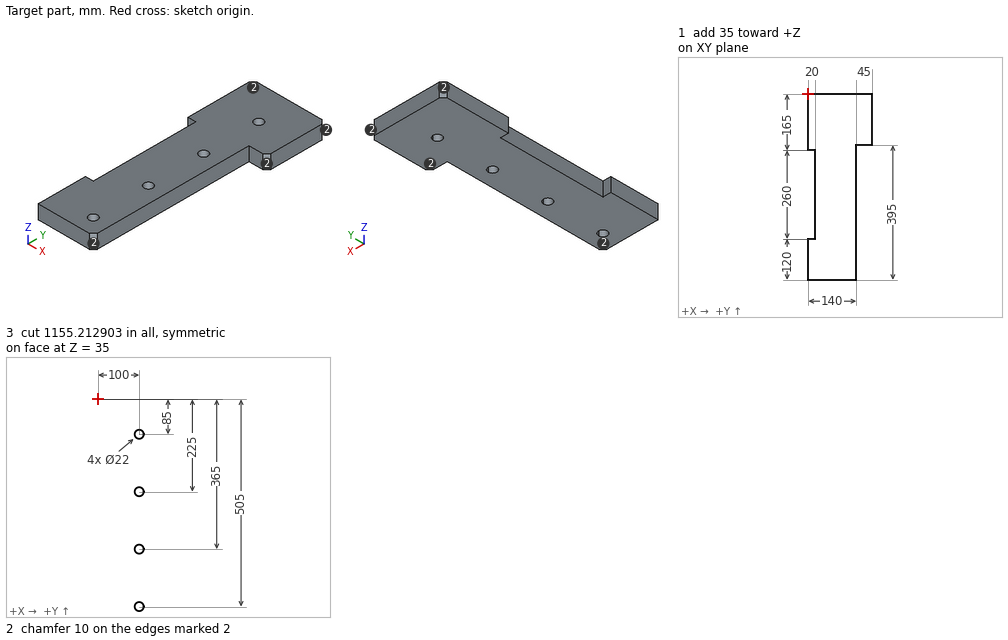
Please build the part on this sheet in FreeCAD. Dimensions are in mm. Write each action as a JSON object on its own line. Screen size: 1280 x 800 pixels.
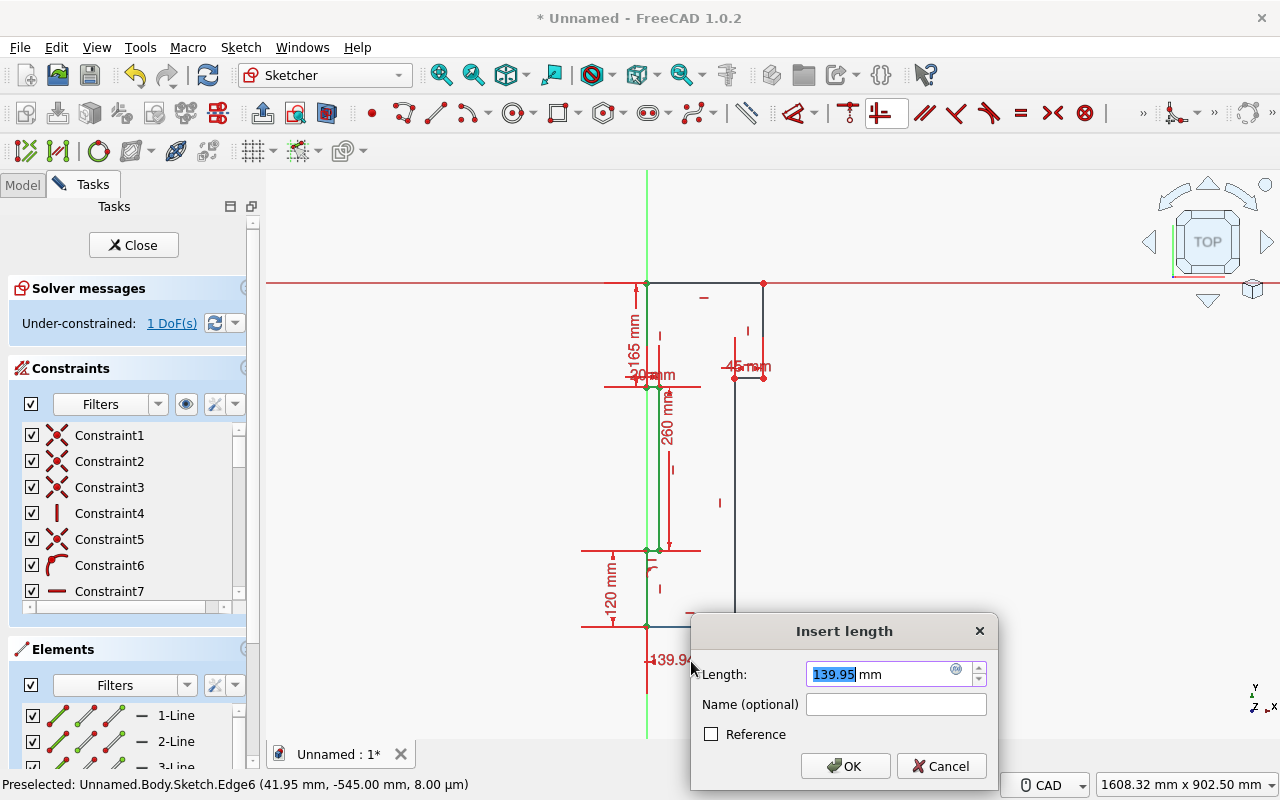
{"action": "type", "text": "140"}
{"action": "key", "text": "Return"}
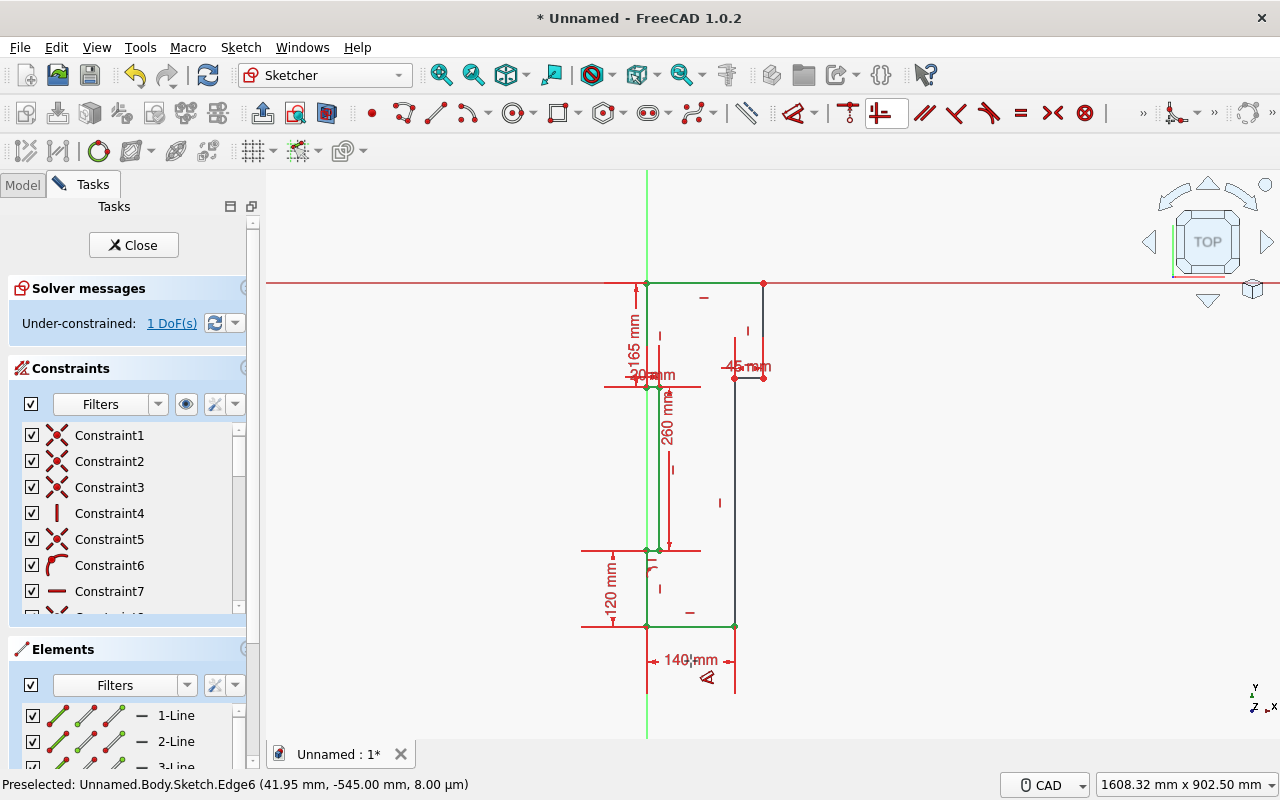
{"action": "left_click", "coordinate": [735, 552]}
{"action": "left_click", "coordinate": [769, 503]}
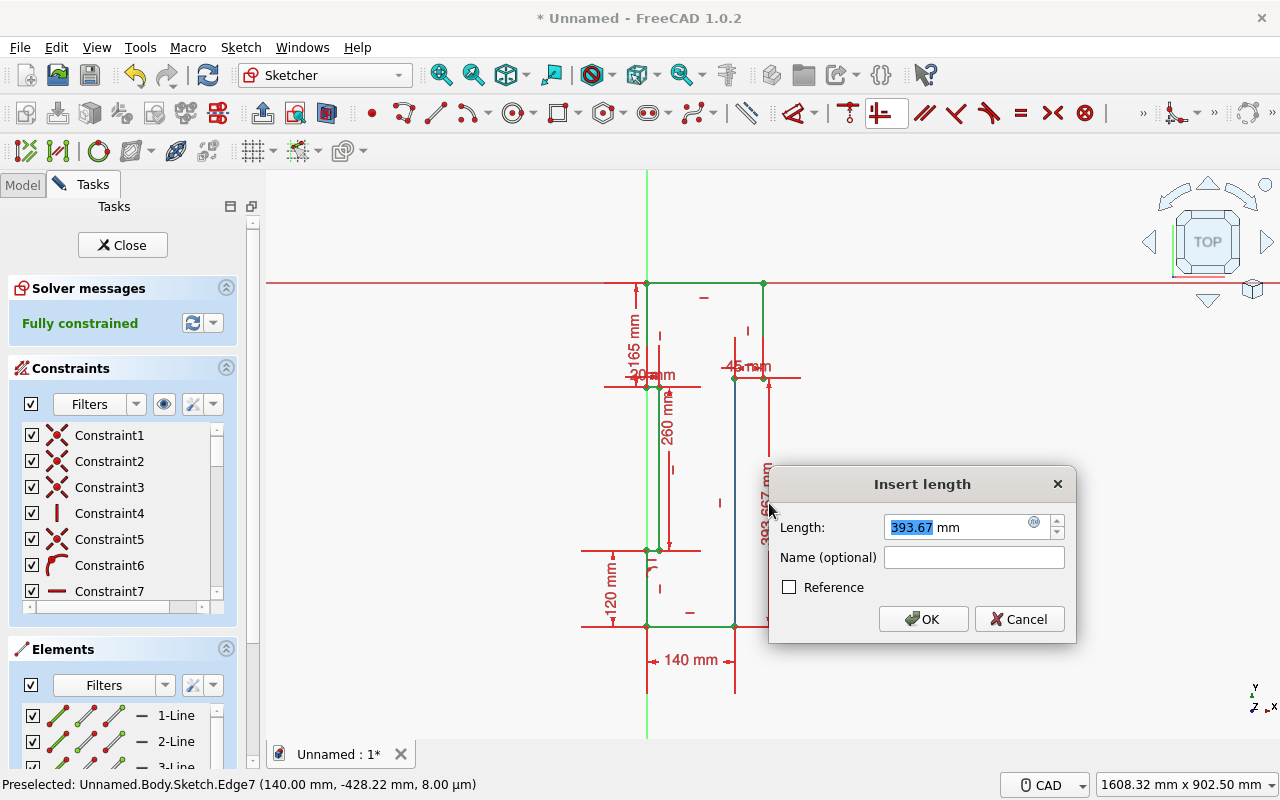
{"action": "type", "text": "395"}
{"action": "key", "text": "Return"}
{"action": "key", "text": "Escape"}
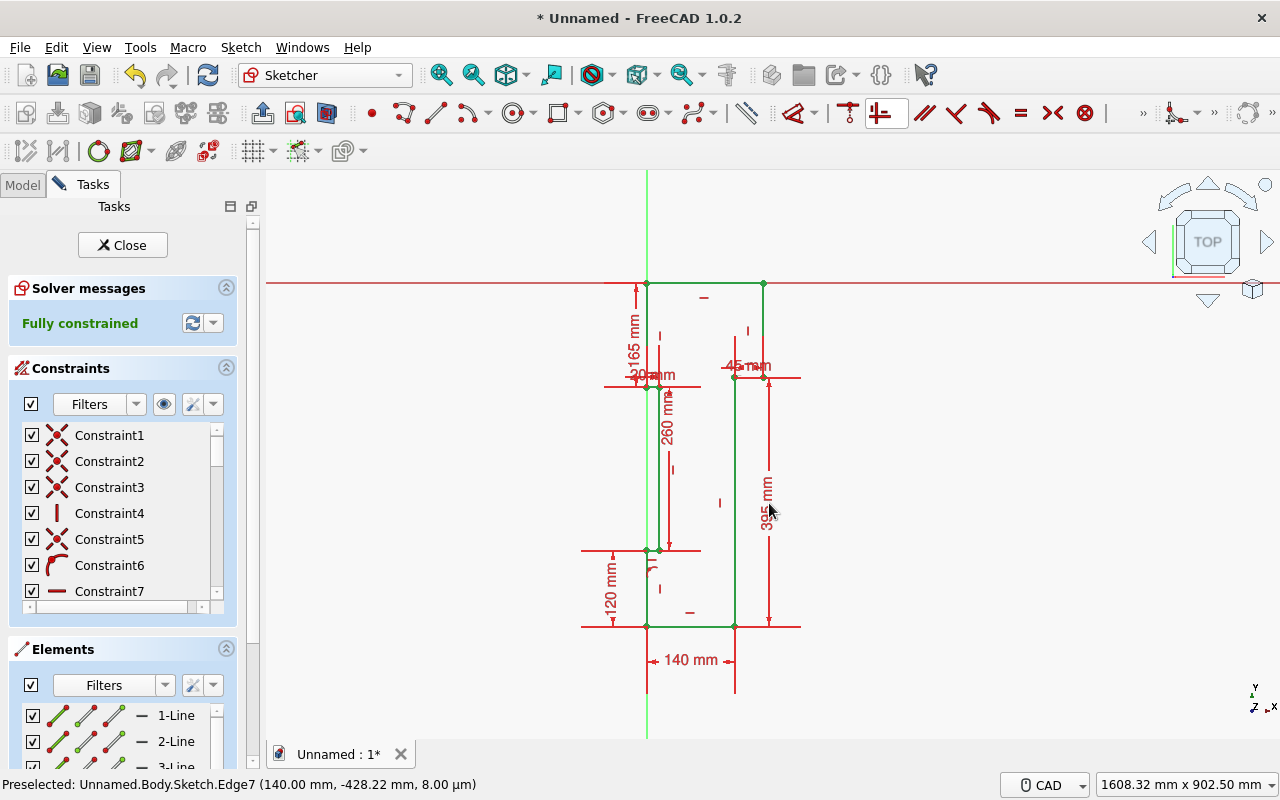
{"action": "left_click", "coordinate": [123, 245]}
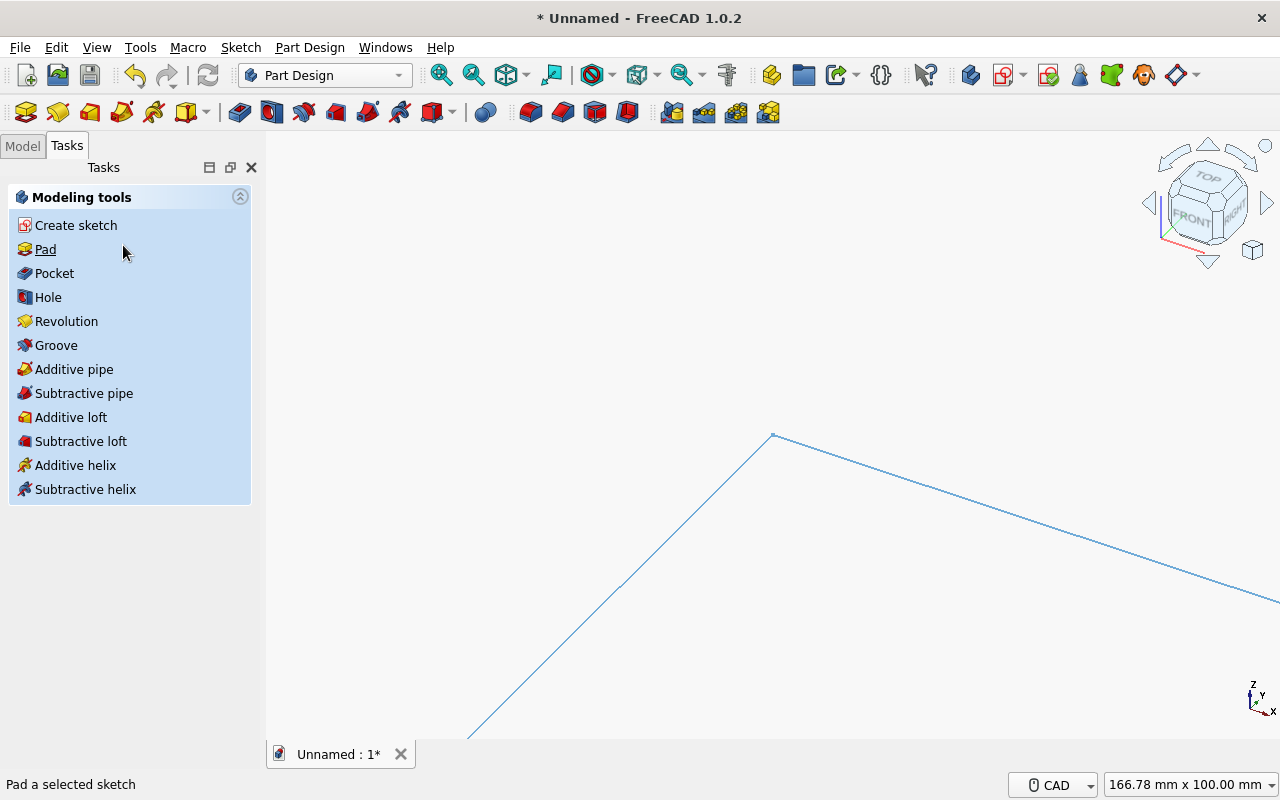
{"action": "left_click", "coordinate": [26, 112]}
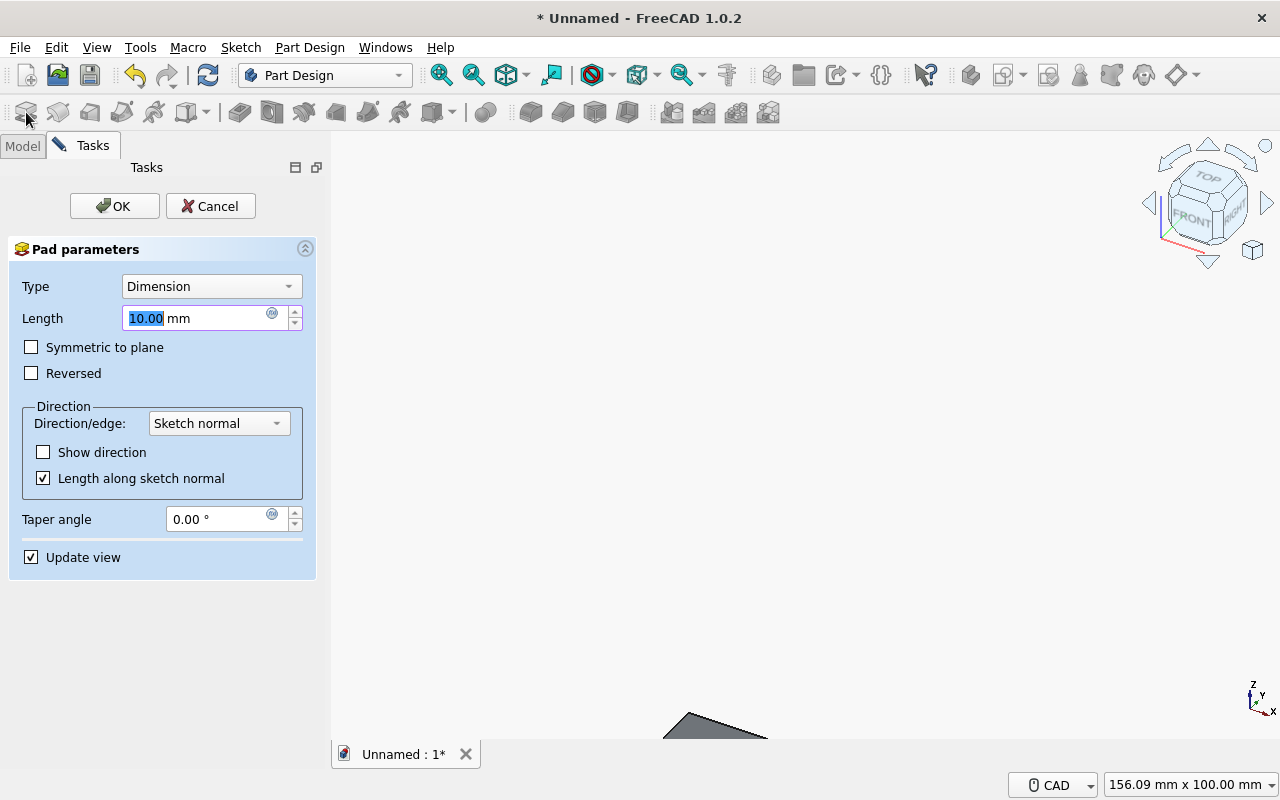
{"action": "type", "text": "35"}
{"action": "key", "text": "Tab"}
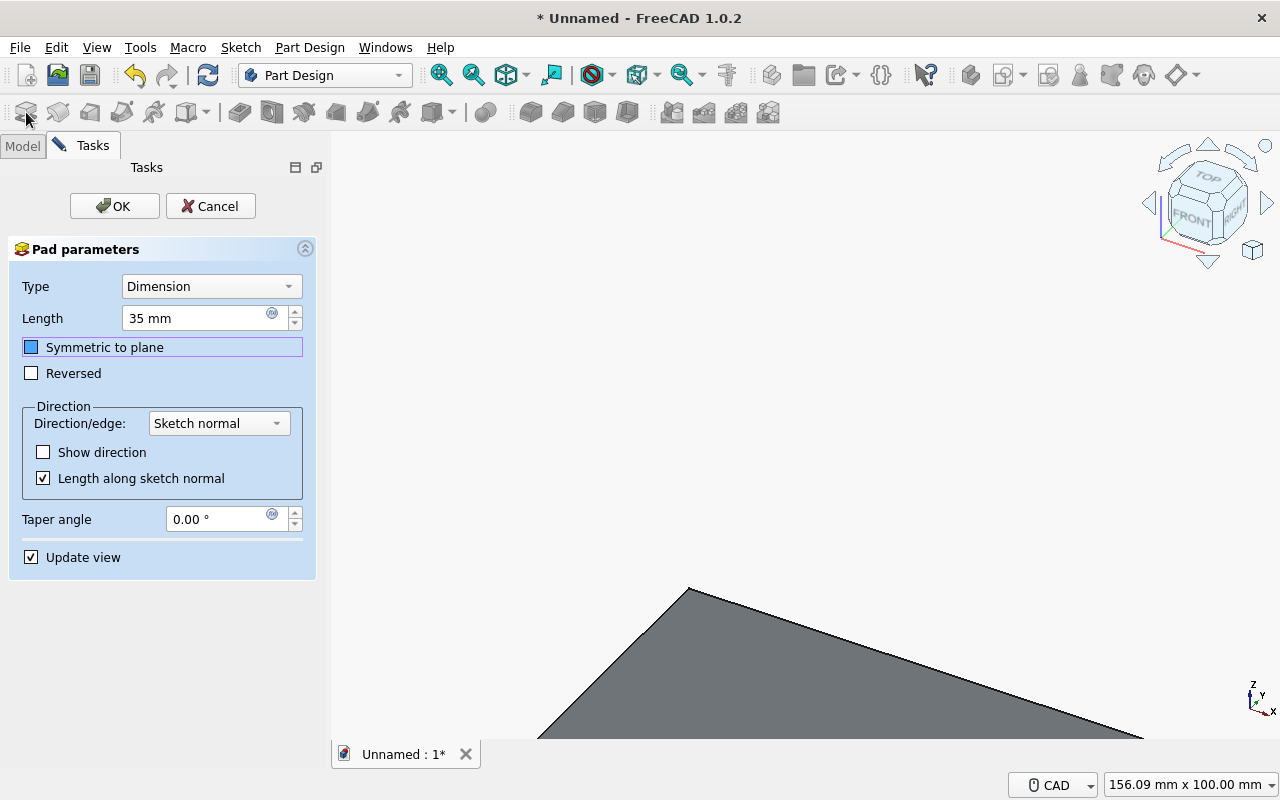
{"action": "left_click", "coordinate": [115, 206]}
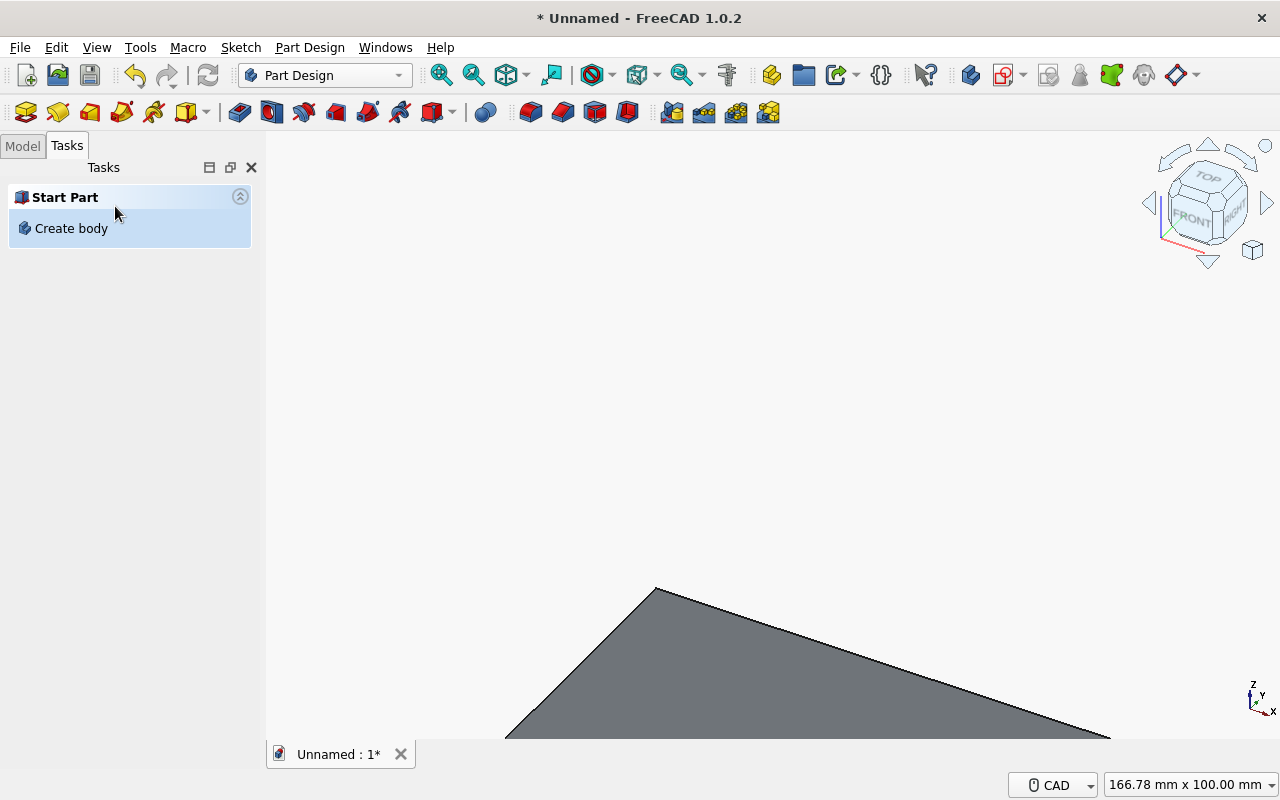
{"action": "left_click", "coordinate": [442, 76]}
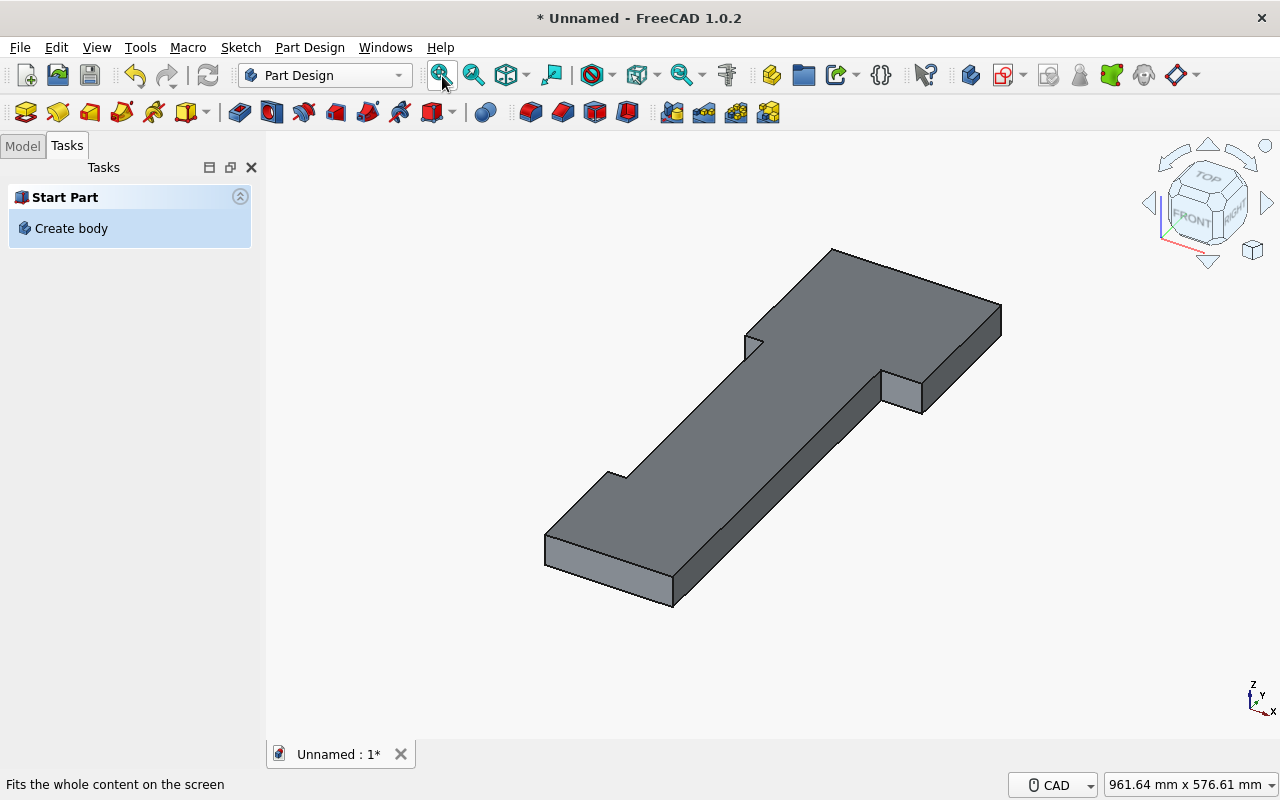
{"action": "left_click", "coordinate": [673, 591]}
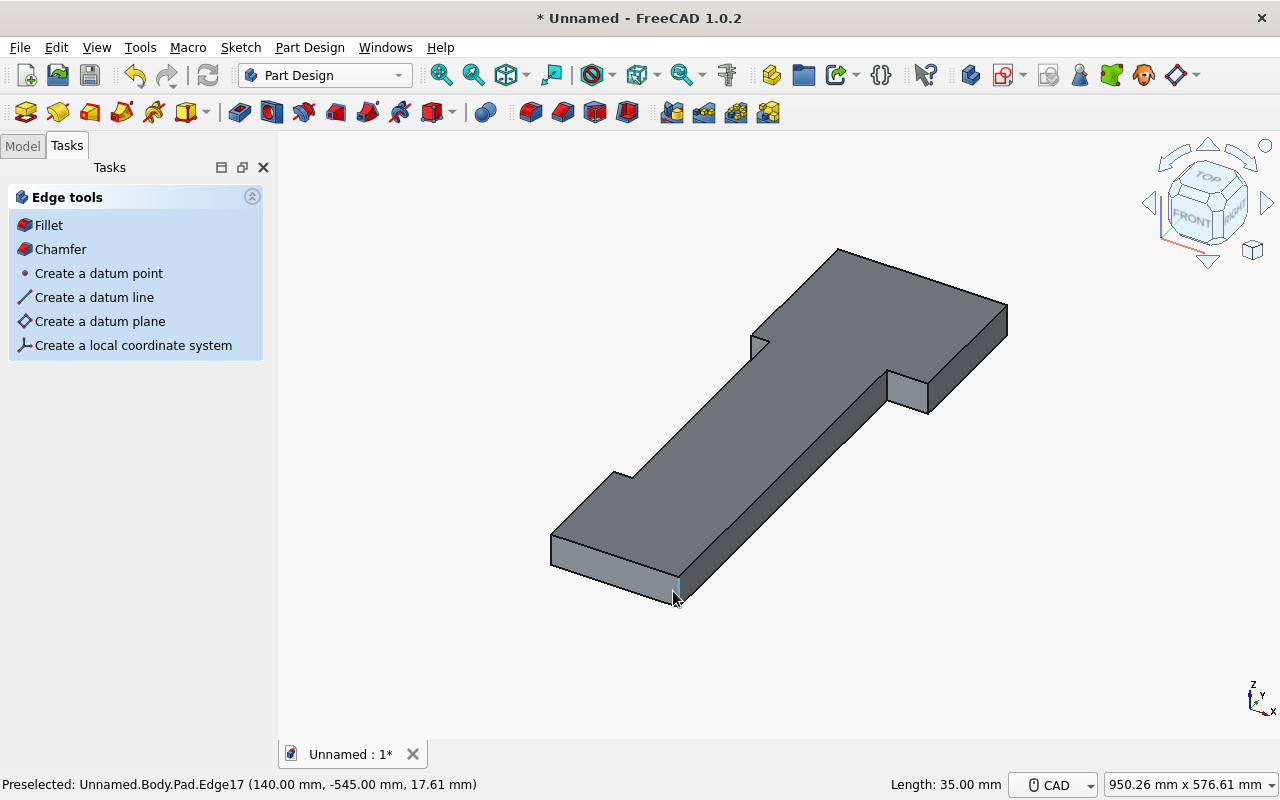
{"action": "left_click", "coordinate": [928, 398], "text": "ctrl"}